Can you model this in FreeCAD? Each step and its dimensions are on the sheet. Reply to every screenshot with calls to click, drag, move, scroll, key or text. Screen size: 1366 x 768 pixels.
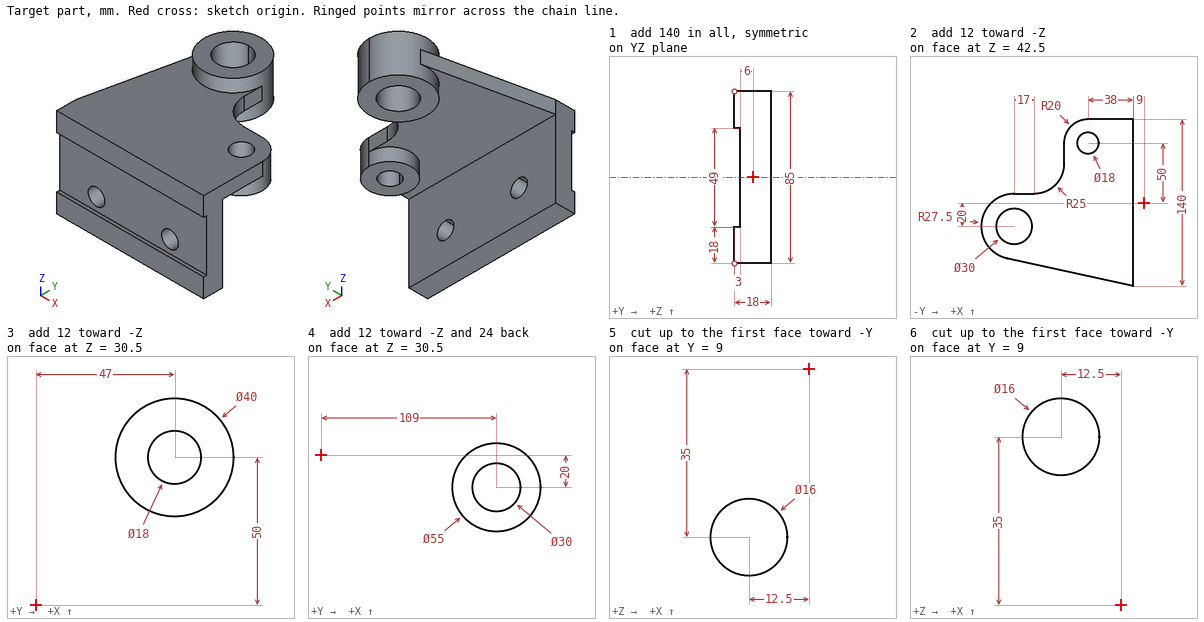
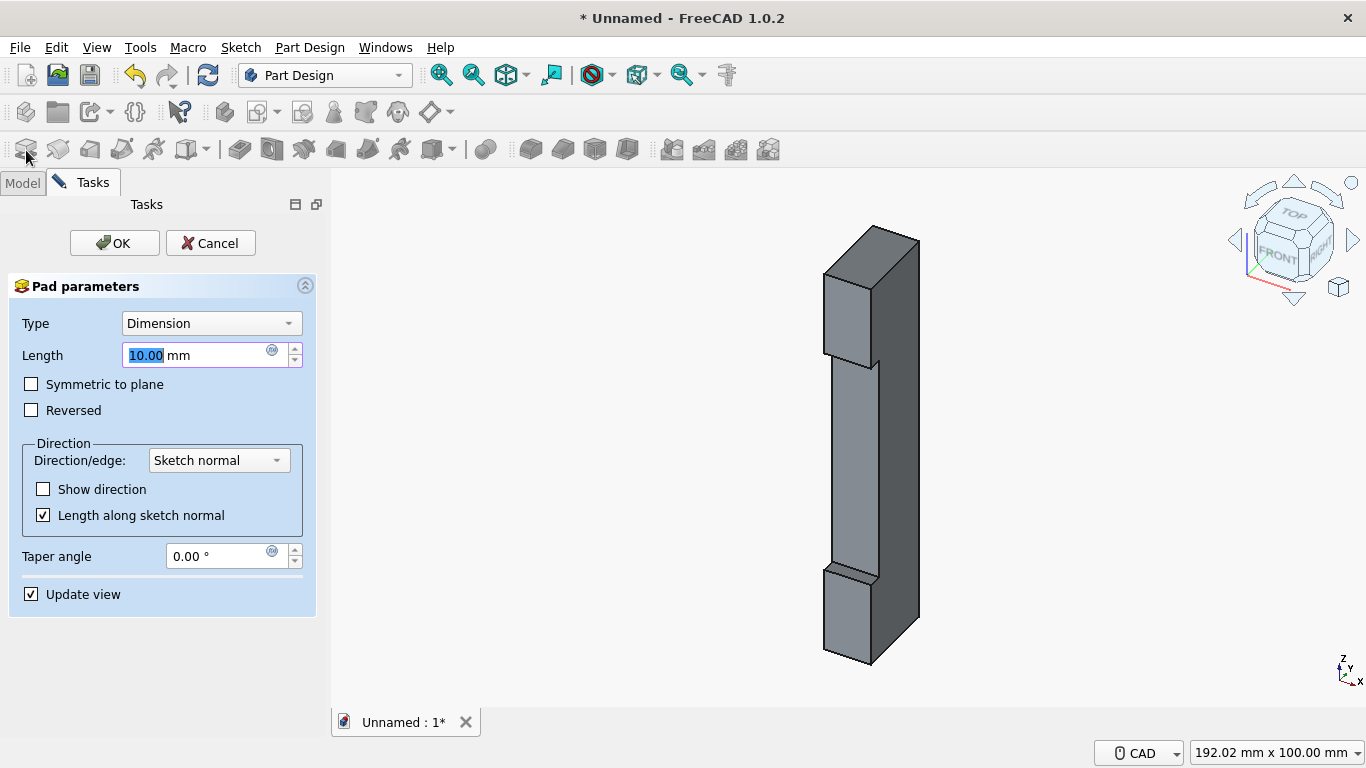
text(140)
key(Tab)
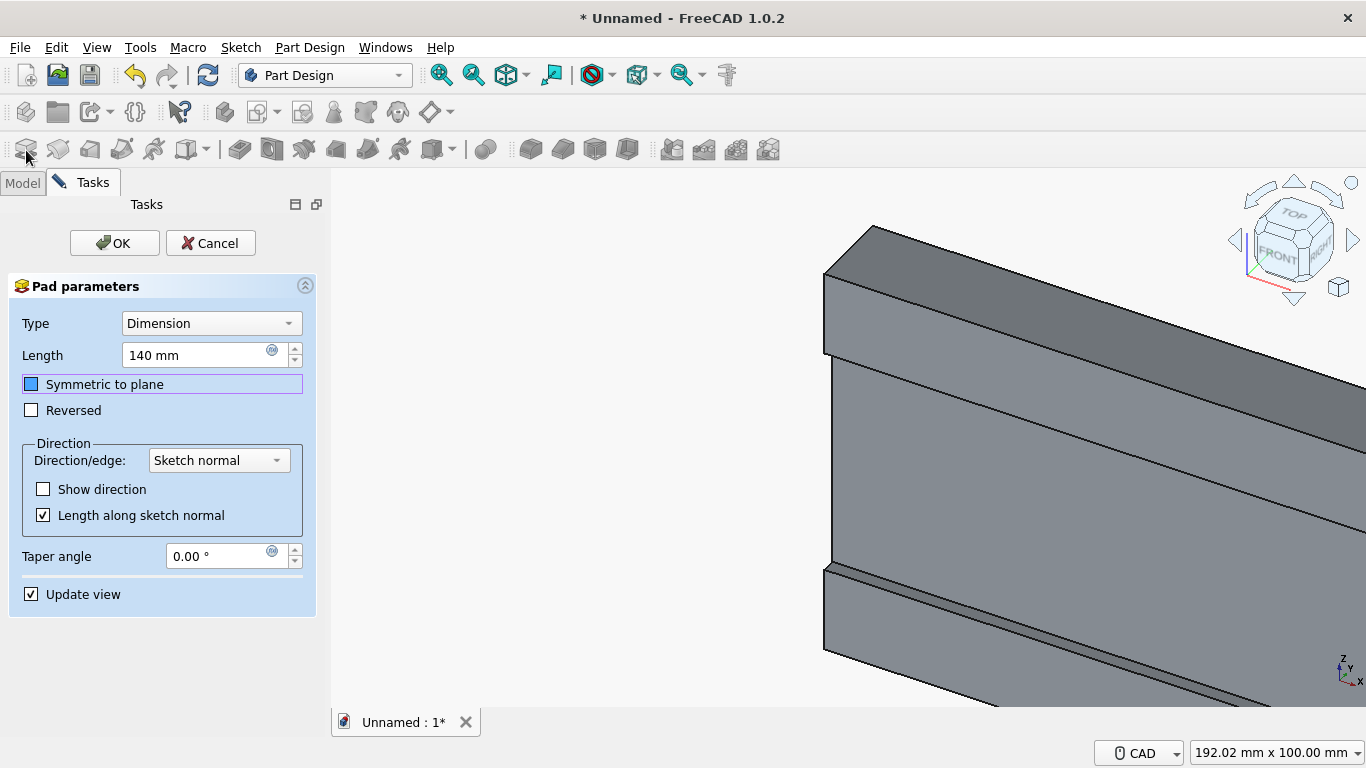
click(30, 384)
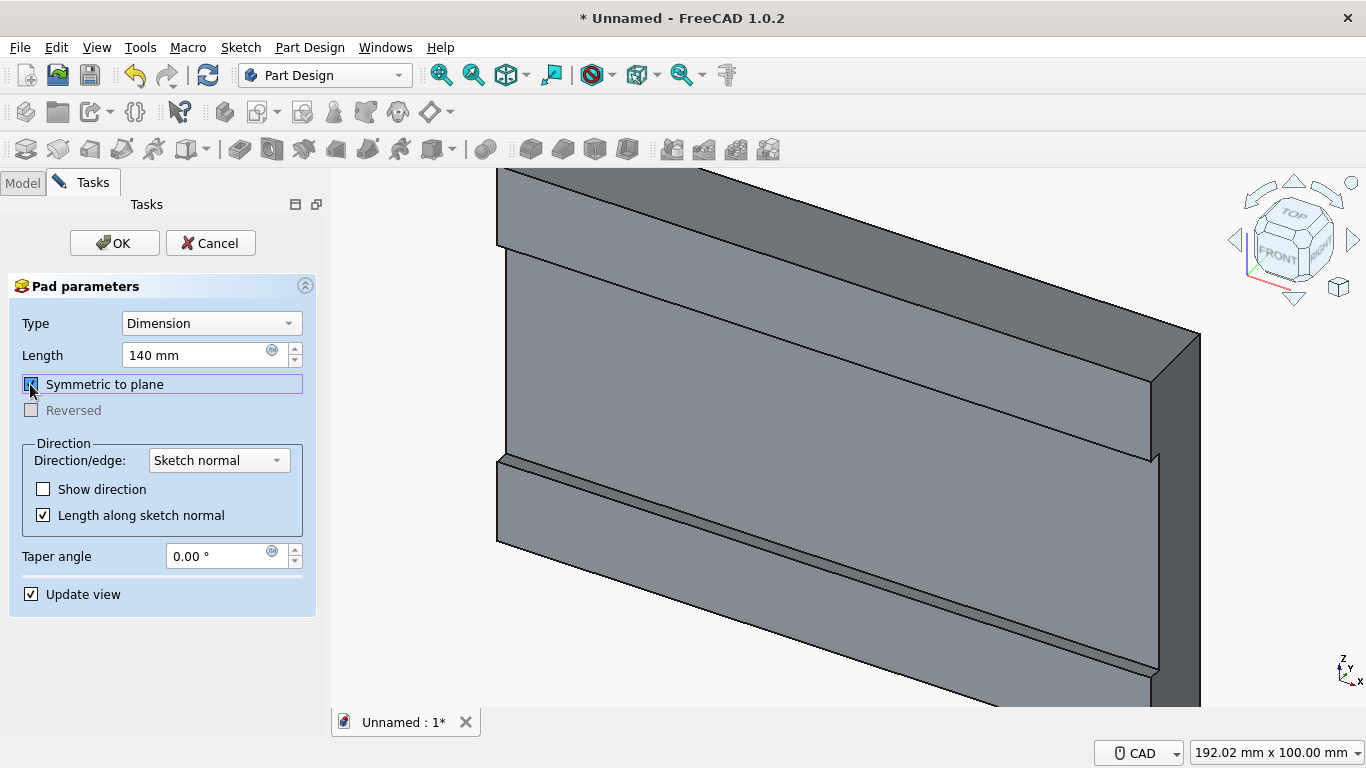
click(115, 243)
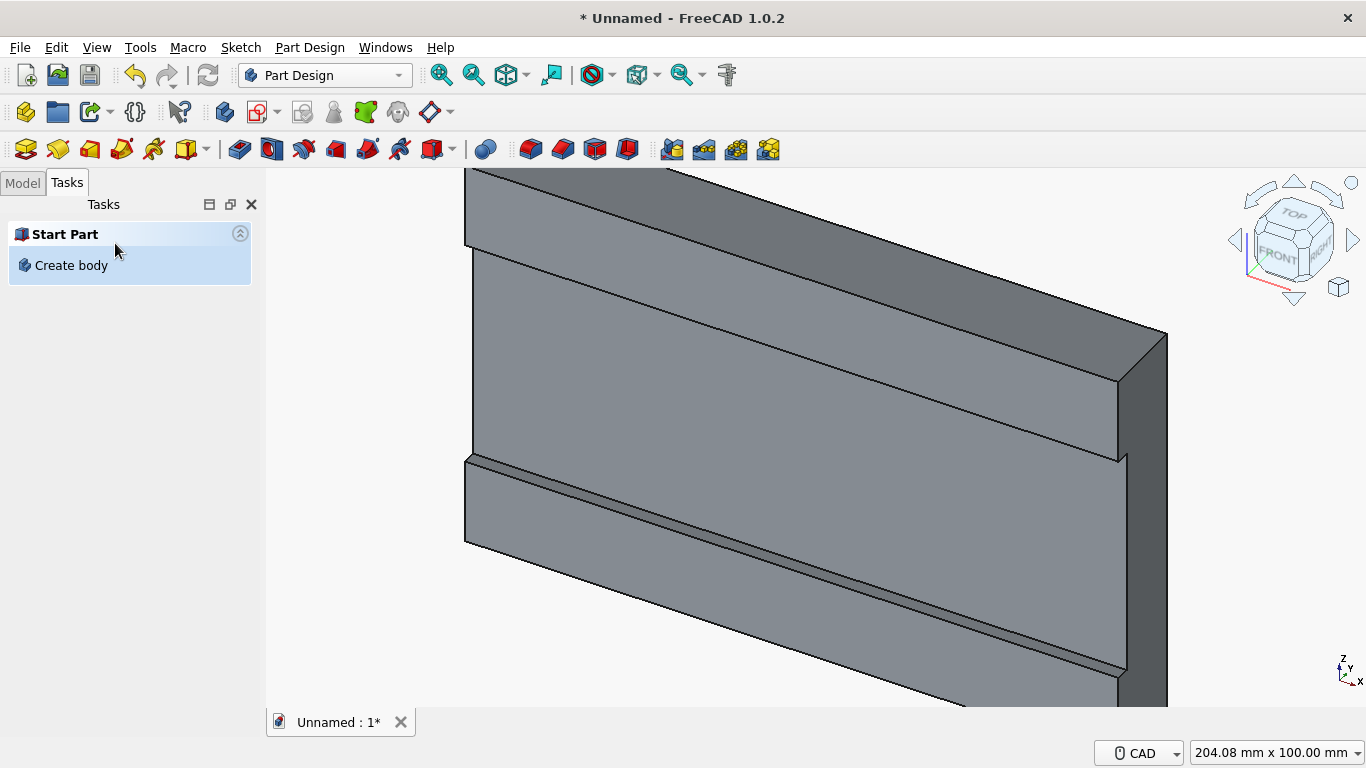
key(v)
key(f)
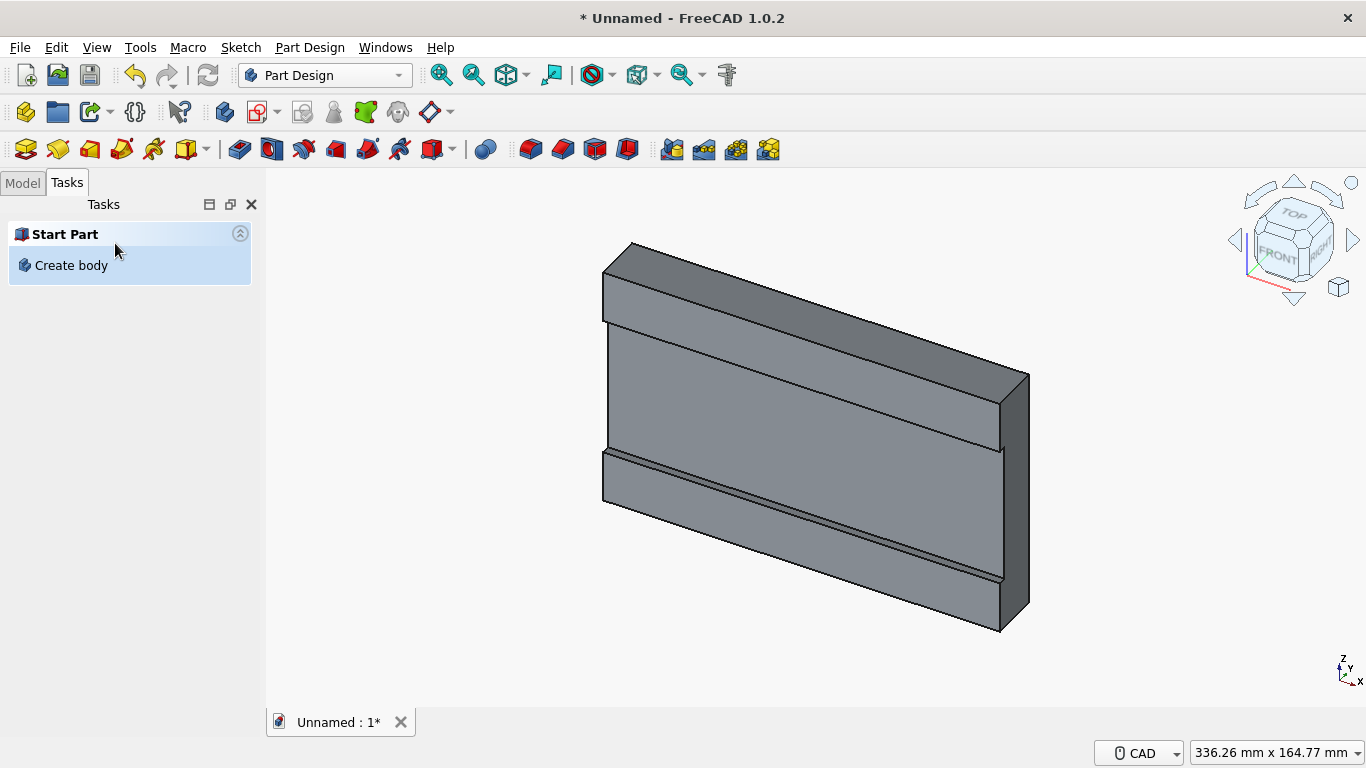
click(816, 323)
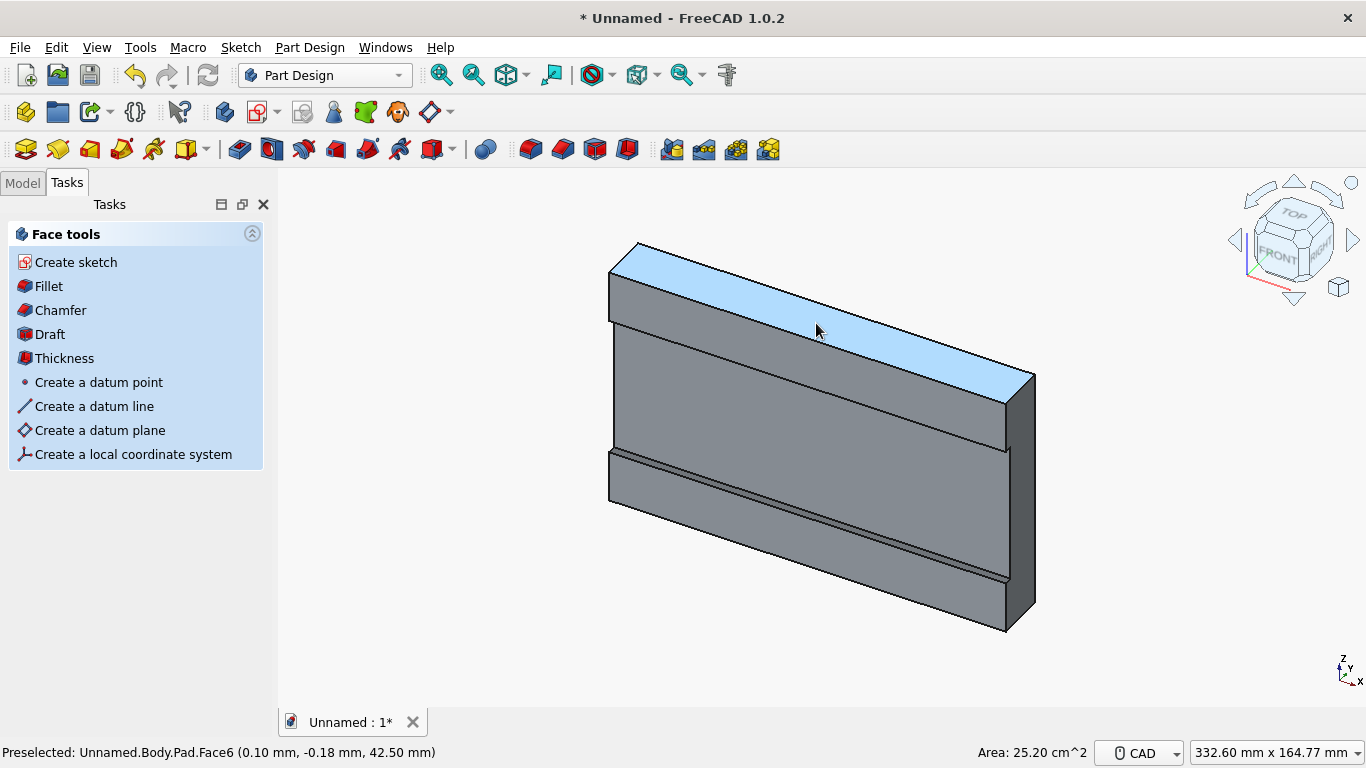
click(258, 112)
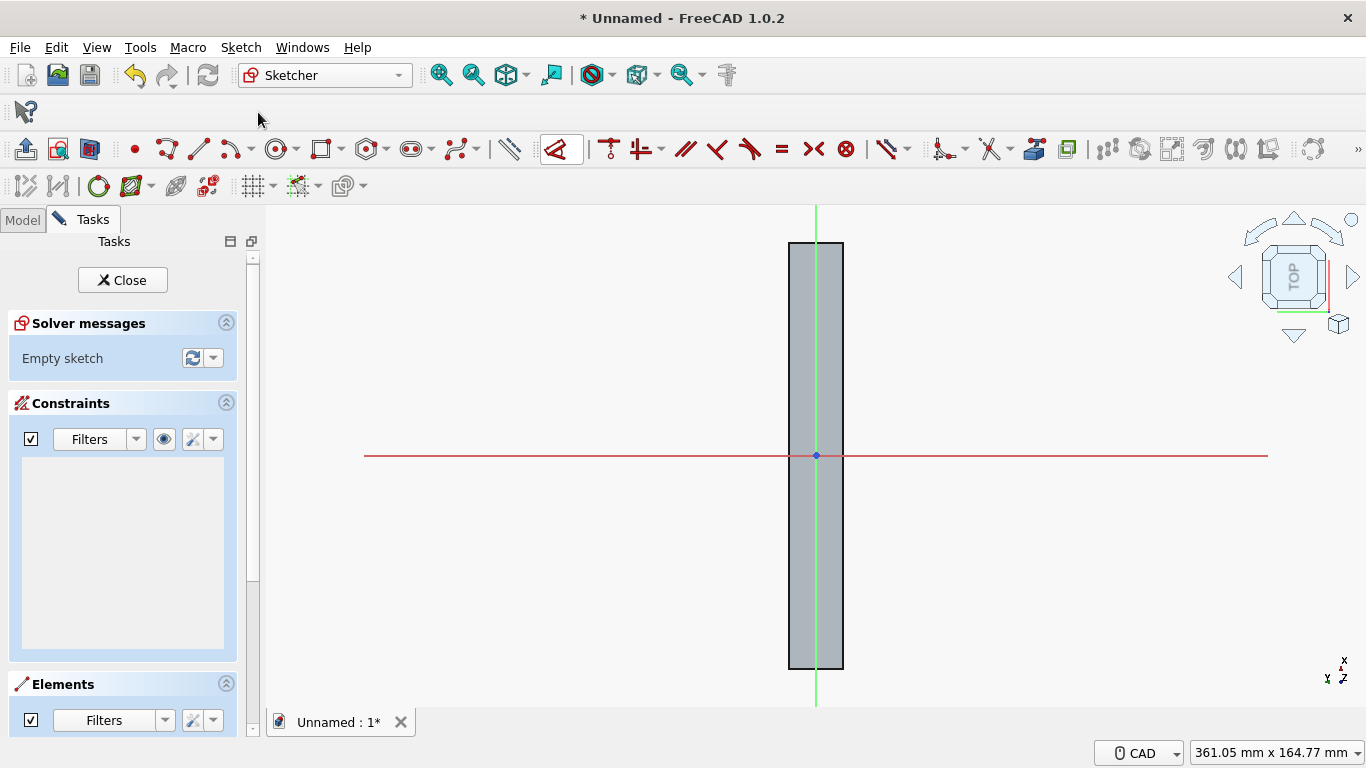
scroll(1031, 456, down, 2)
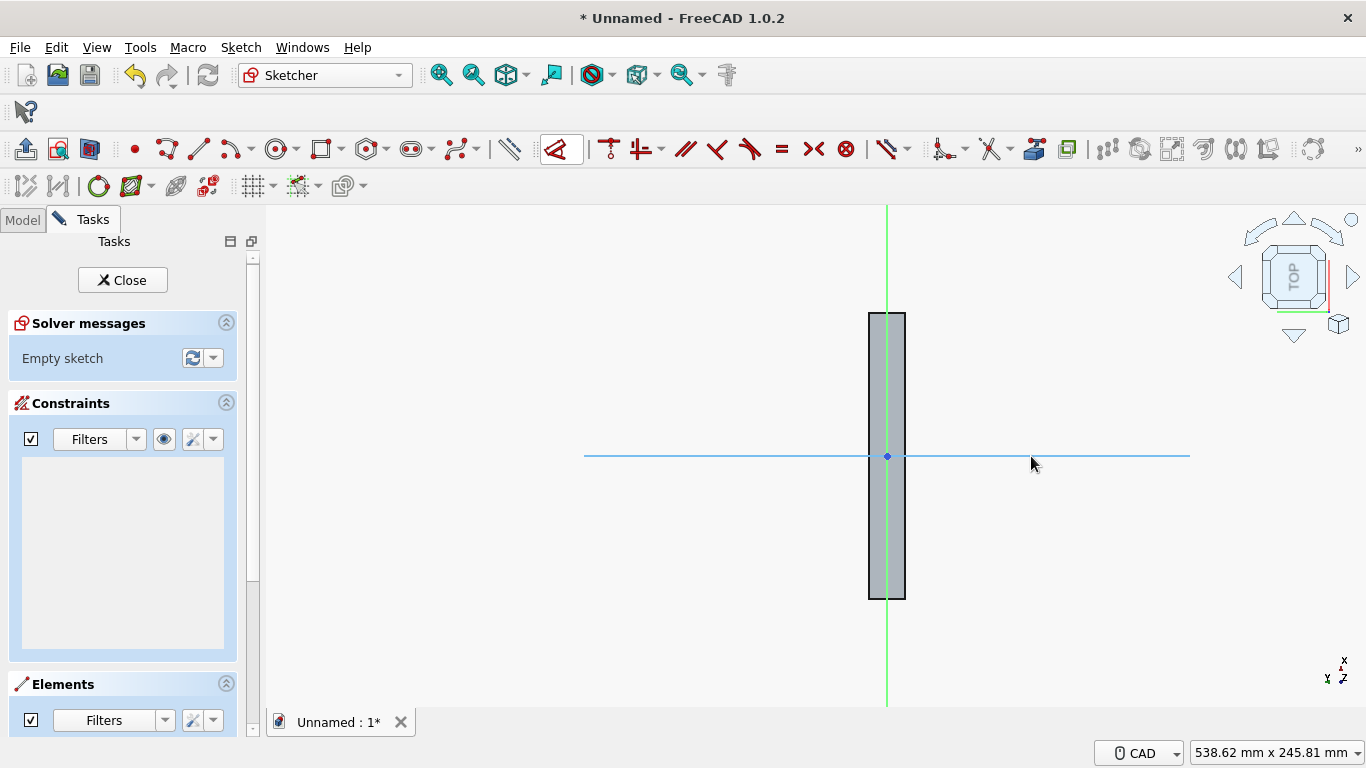
key(g)
key(m)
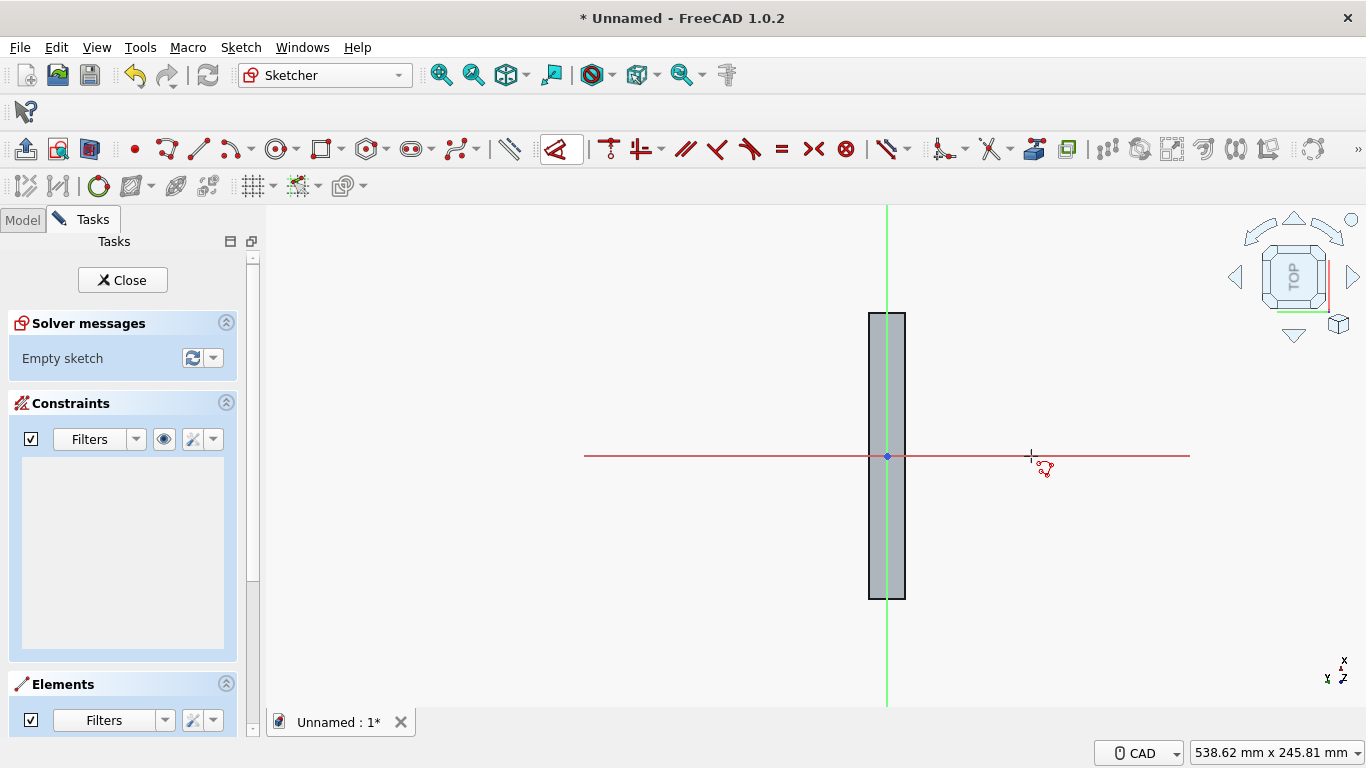
click(791, 313)
click(869, 313)
click(869, 599)
click(653, 552)
right_click(653, 552)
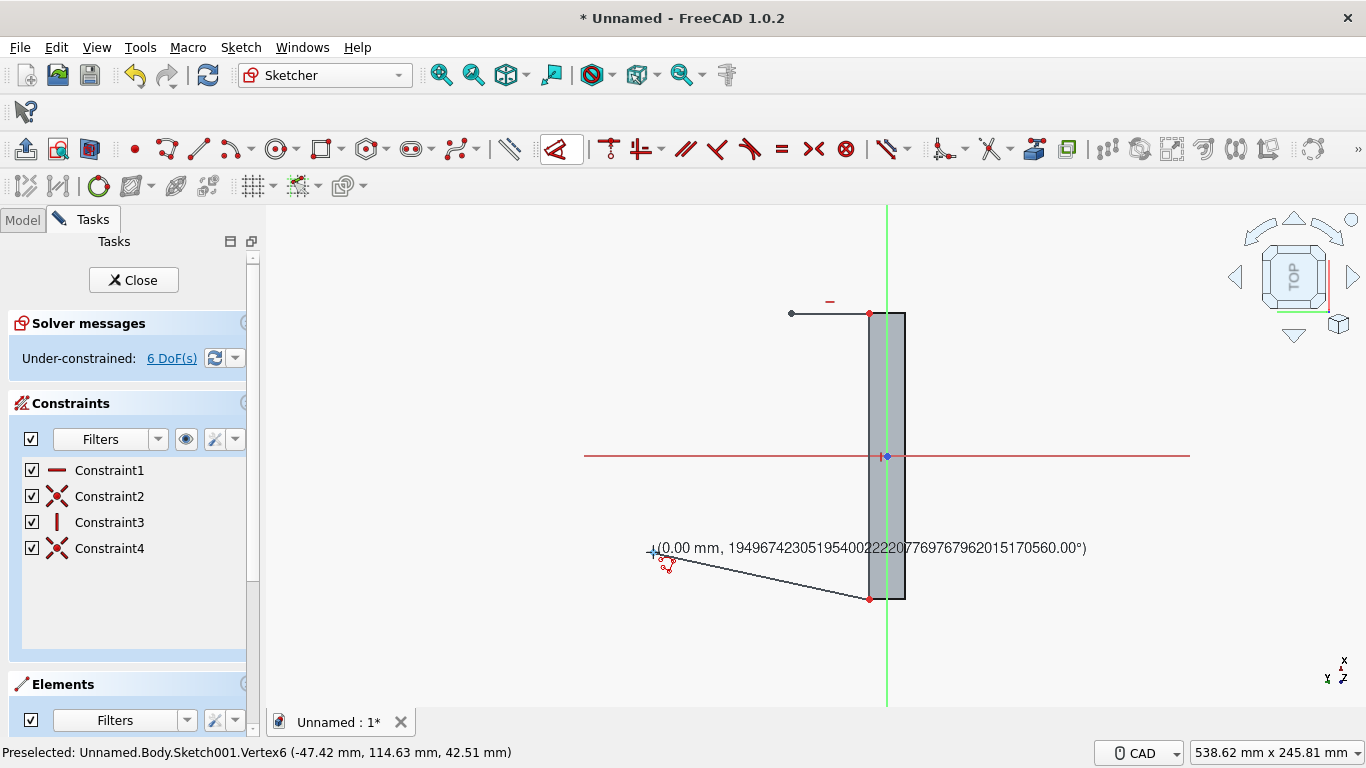
click(200, 150)